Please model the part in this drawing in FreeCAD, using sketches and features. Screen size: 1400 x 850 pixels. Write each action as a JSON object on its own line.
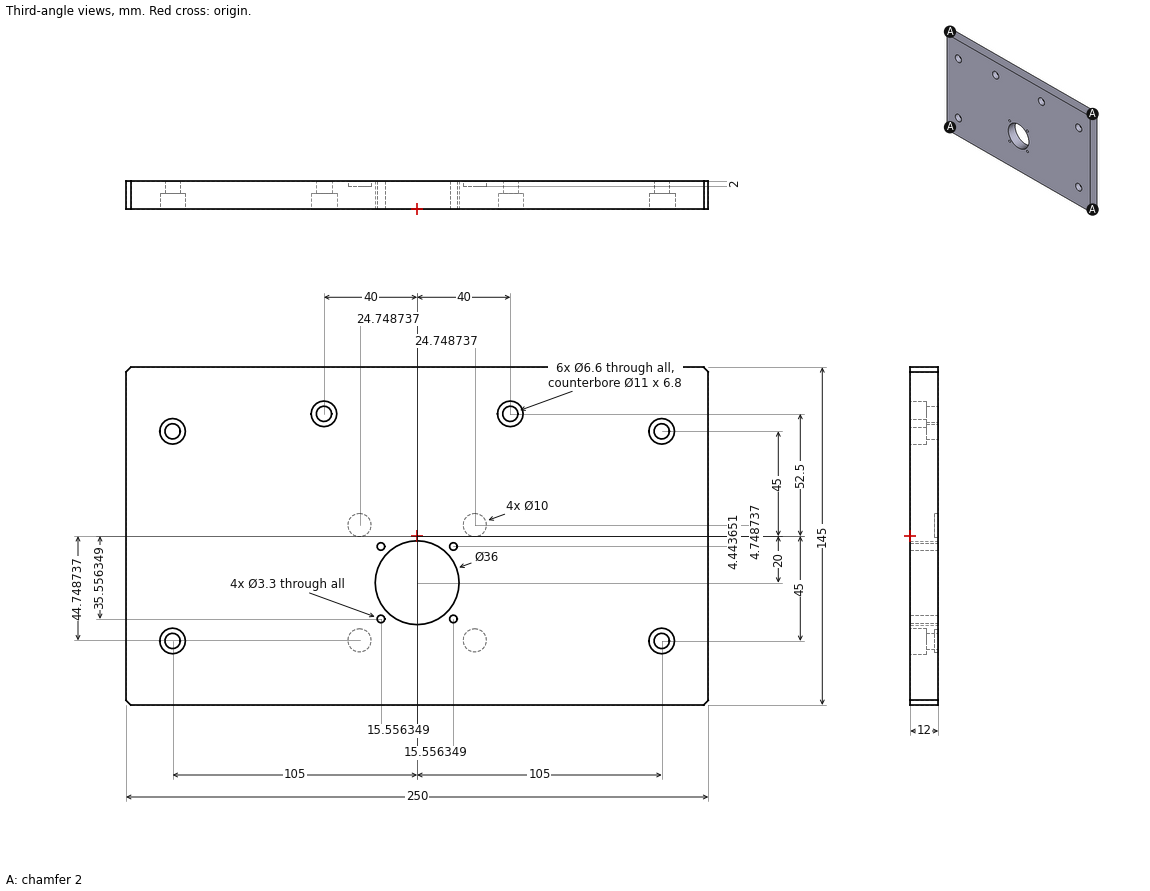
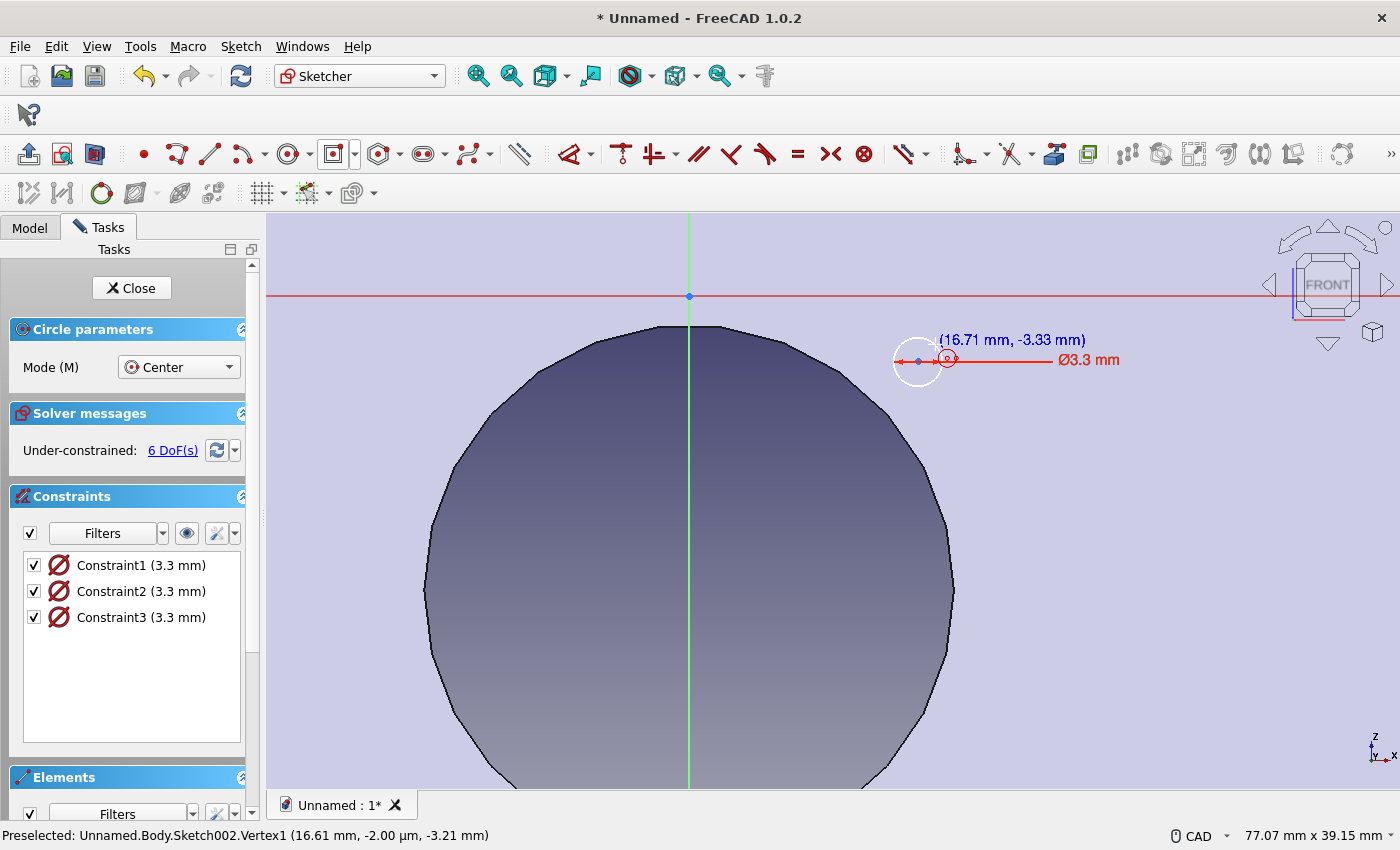
{"action": "left_click", "coordinate": [460, 361]}
{"action": "mouse_move", "coordinate": [477, 344]}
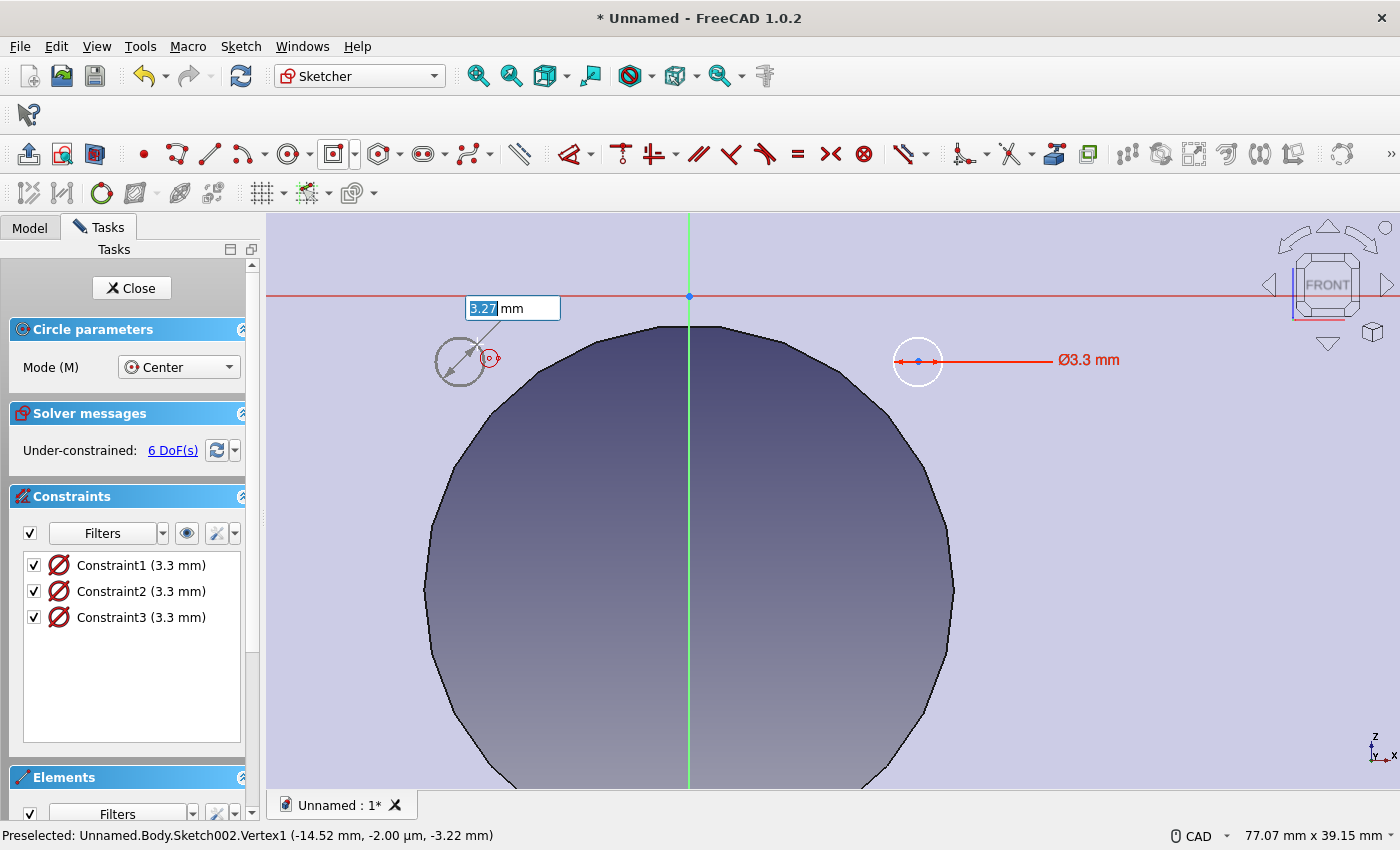
{"action": "type", "text": "3.3"}
{"action": "key", "text": "Return"}
{"action": "key", "text": "Escape"}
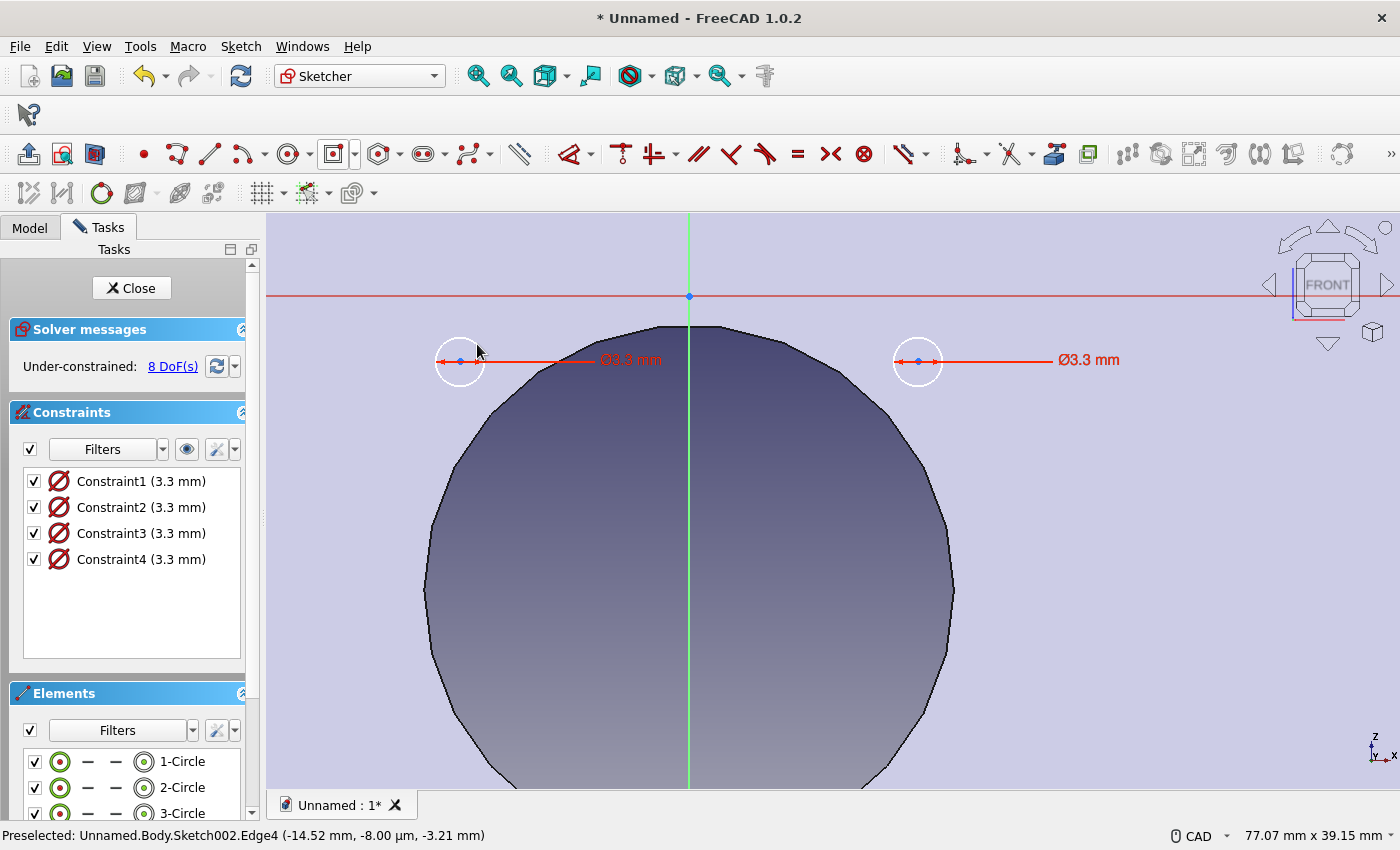
{"action": "scroll", "coordinate": [918, 361], "scroll_direction": "down", "scroll_amount": 2}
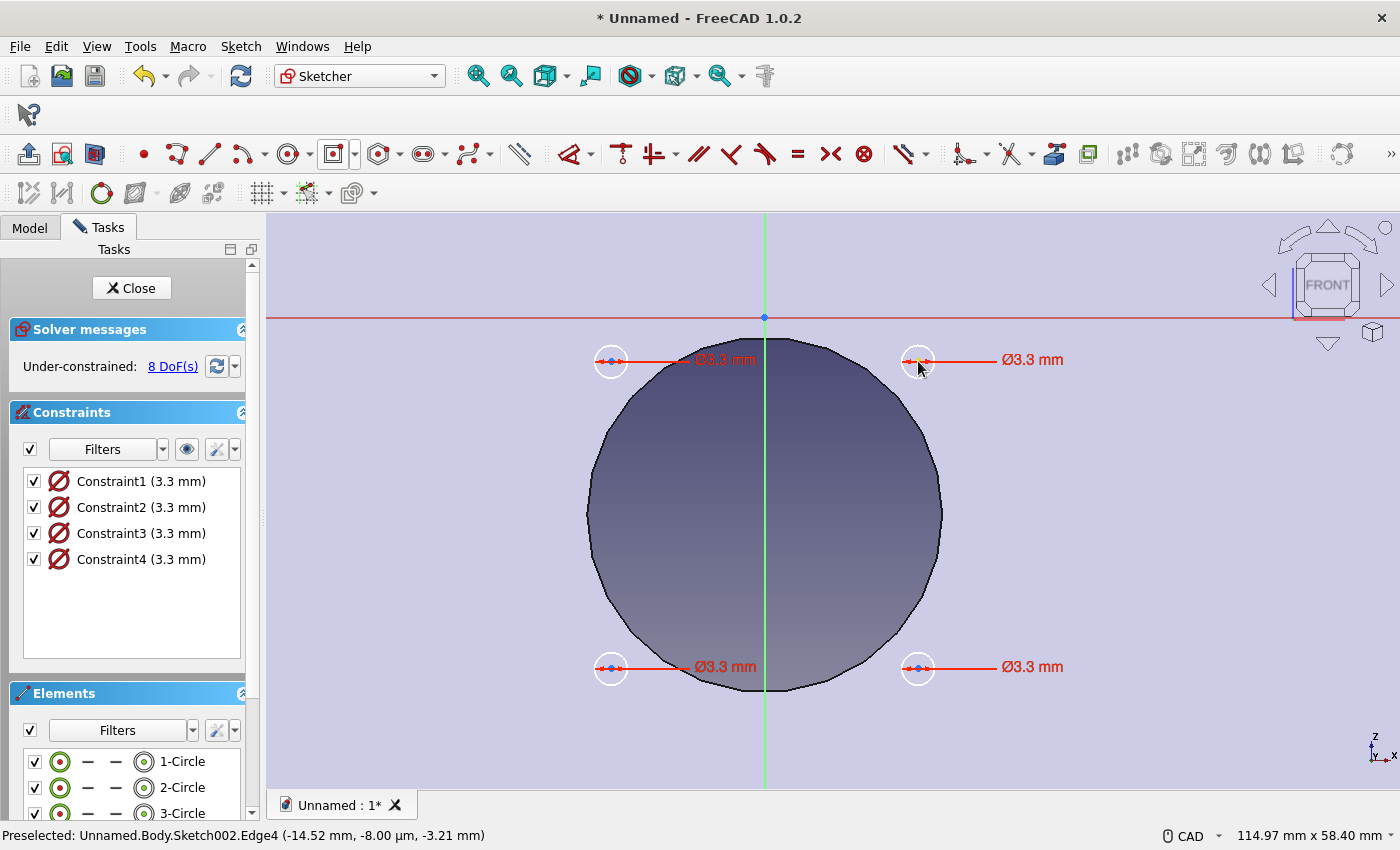
{"action": "left_click", "coordinate": [611, 669]}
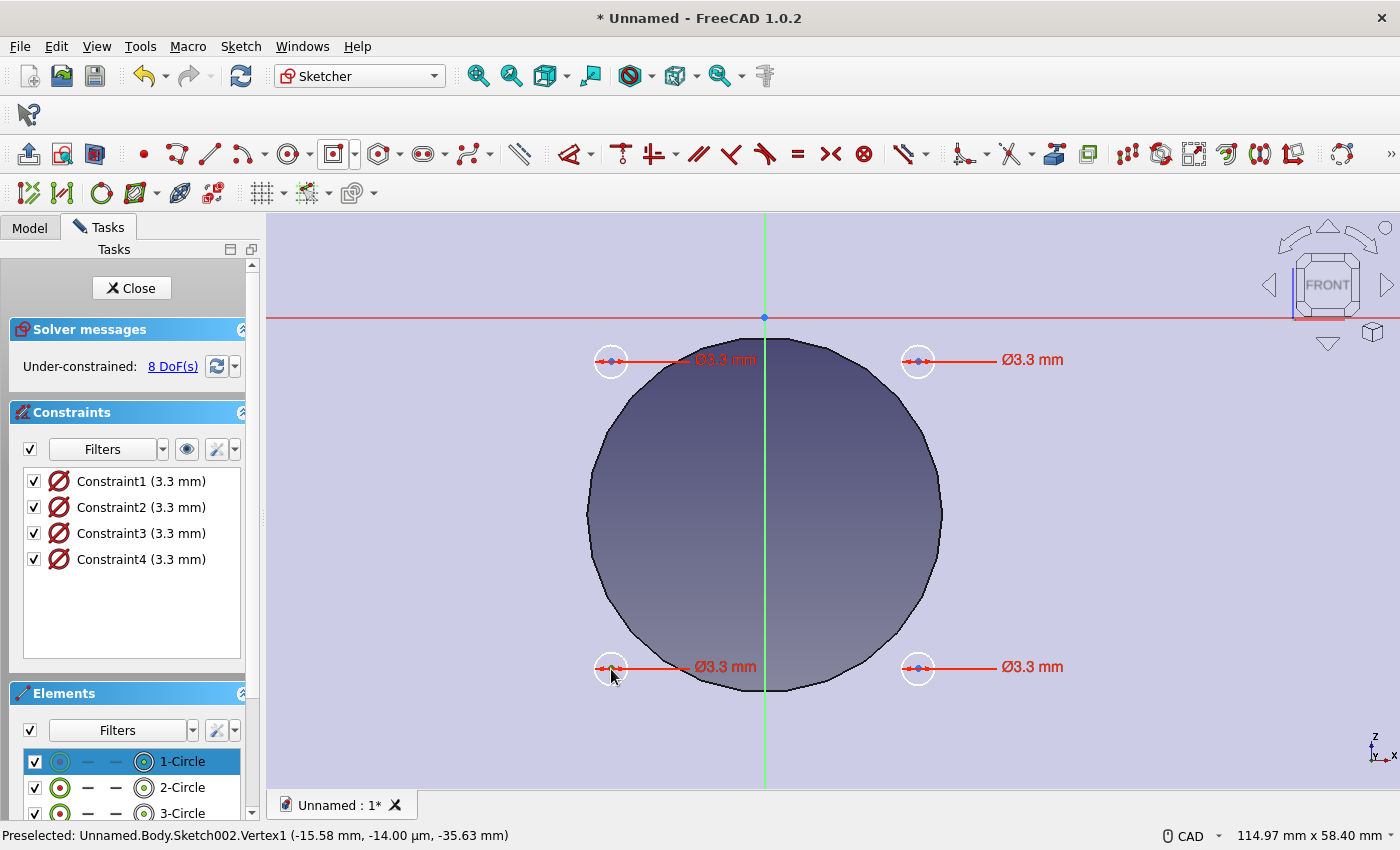
{"action": "left_click", "coordinate": [918, 669]}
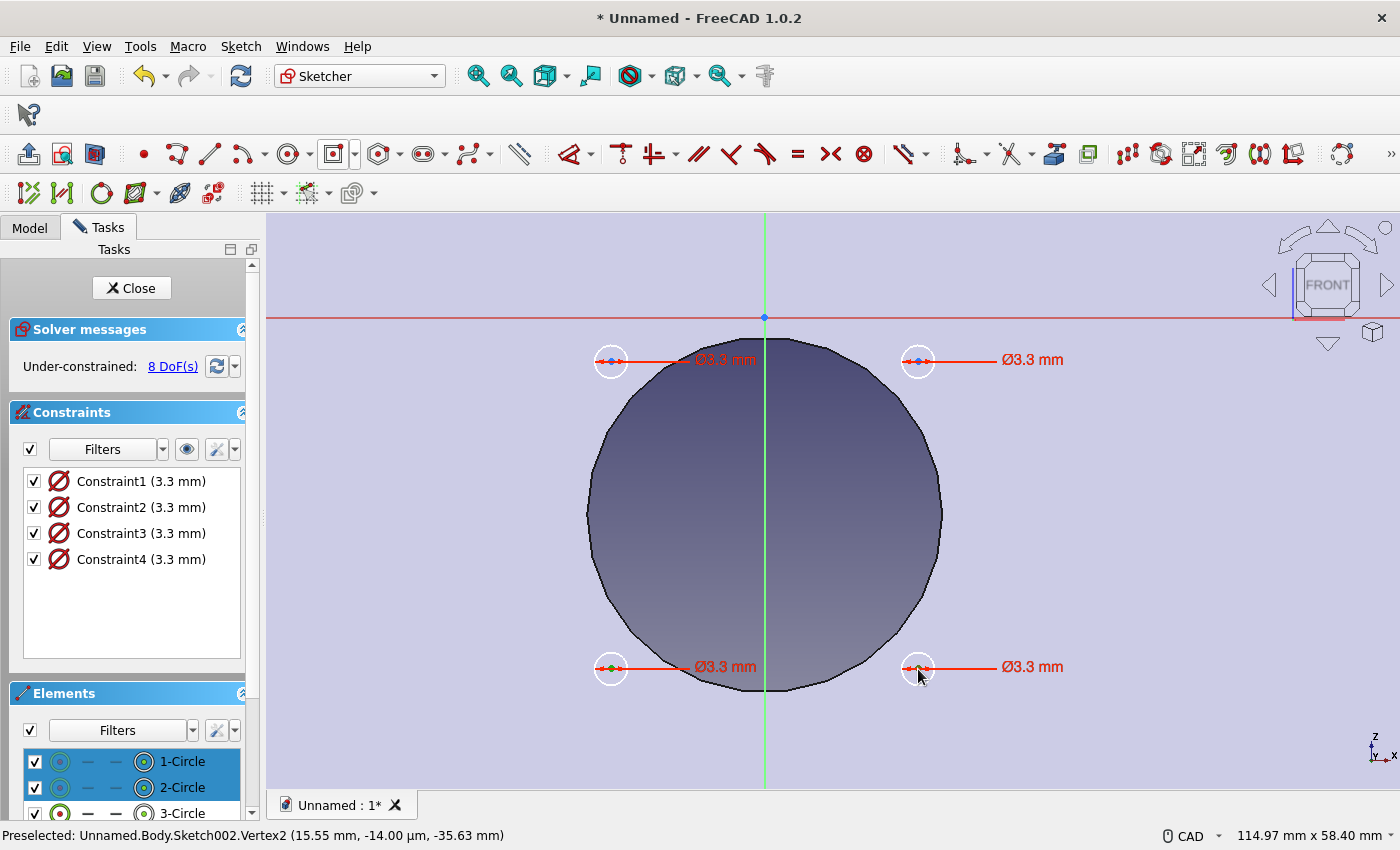
{"action": "left_click", "coordinate": [676, 154]}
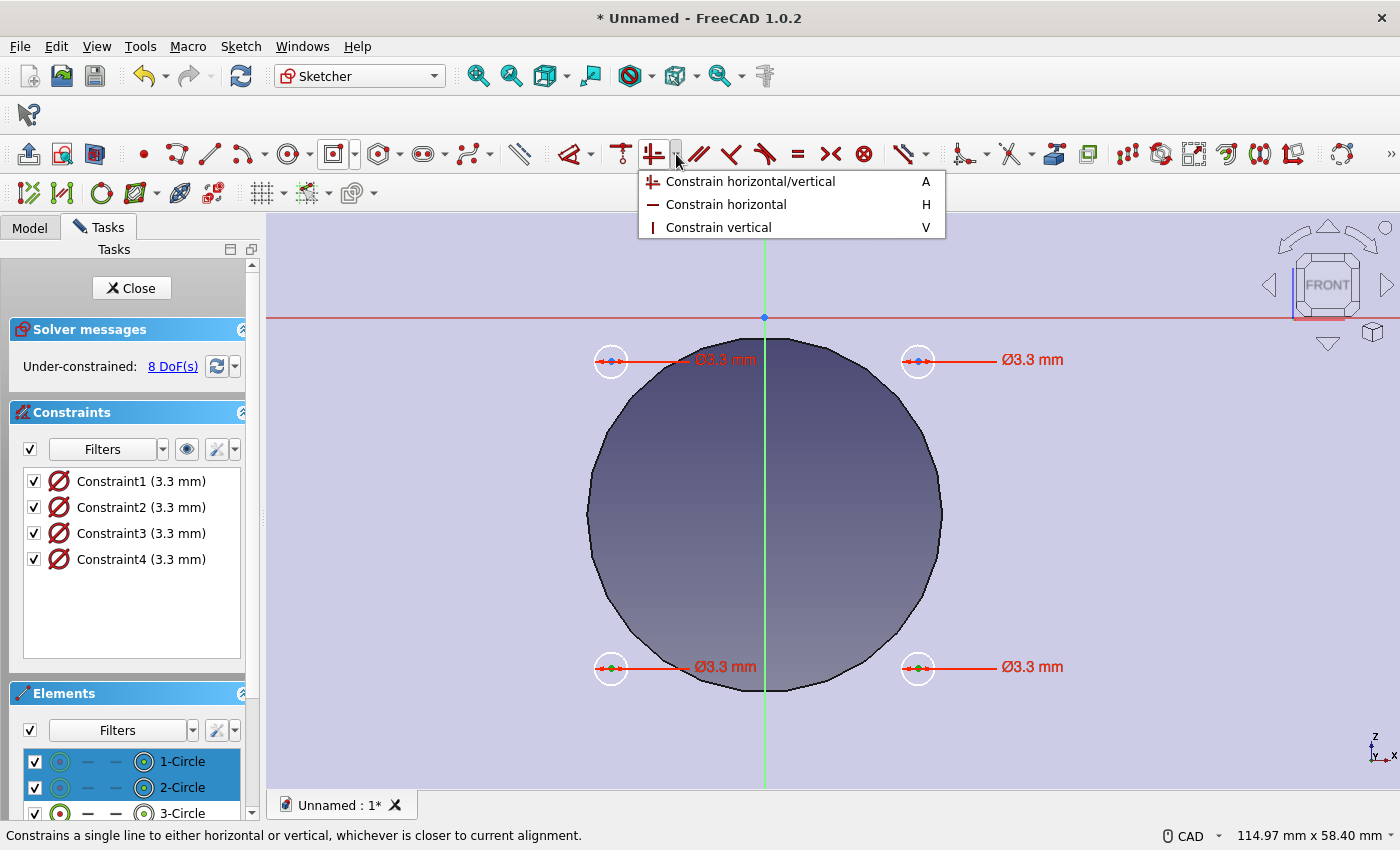
{"action": "left_click", "coordinate": [792, 204]}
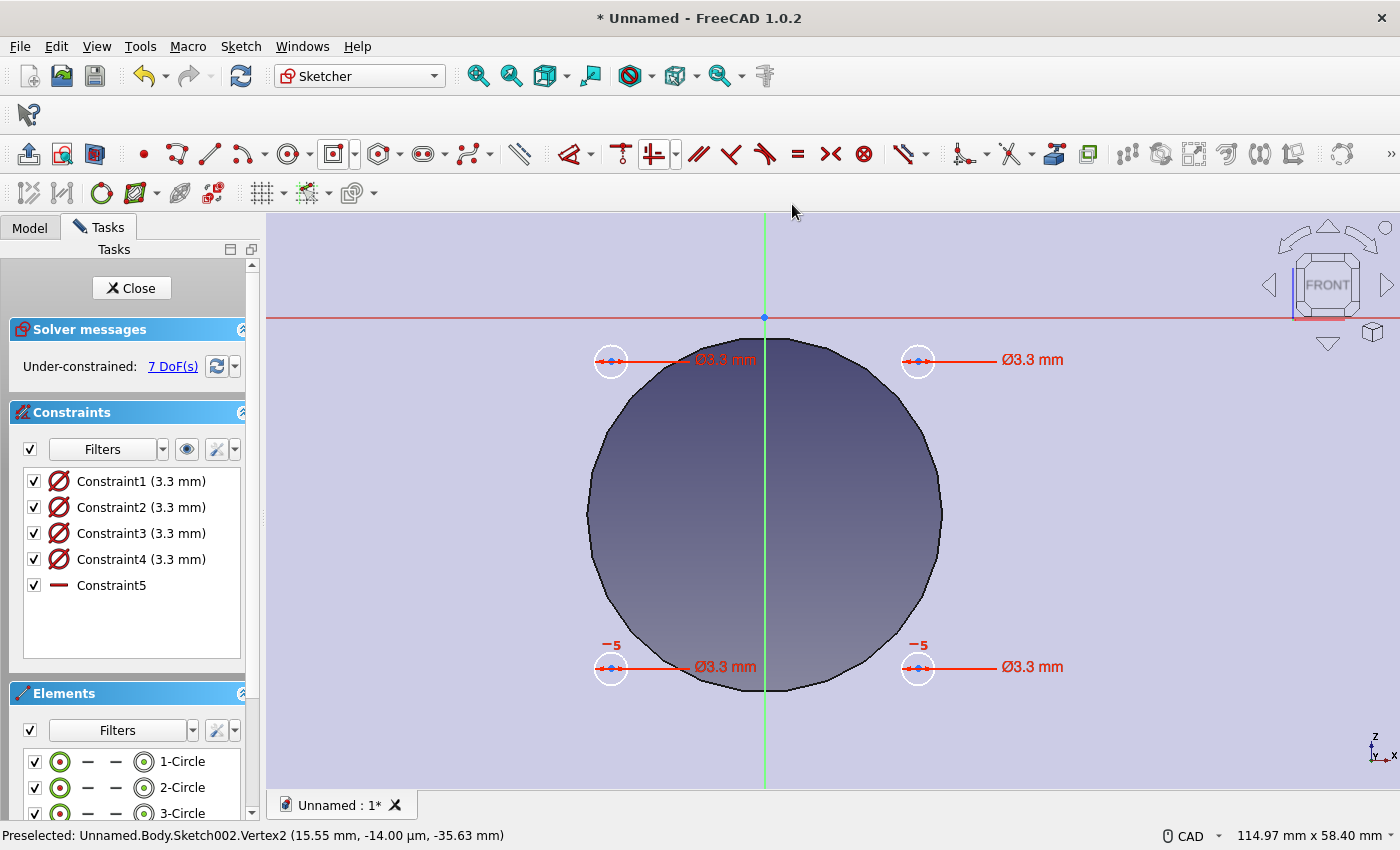
{"action": "left_click", "coordinate": [918, 669]}